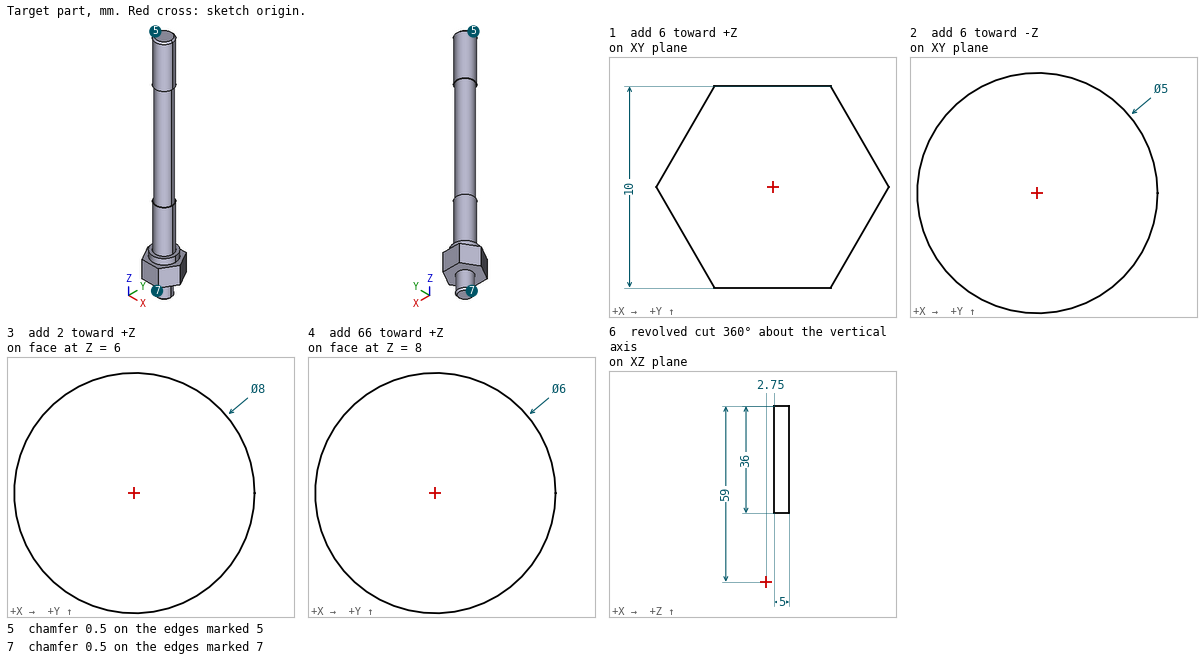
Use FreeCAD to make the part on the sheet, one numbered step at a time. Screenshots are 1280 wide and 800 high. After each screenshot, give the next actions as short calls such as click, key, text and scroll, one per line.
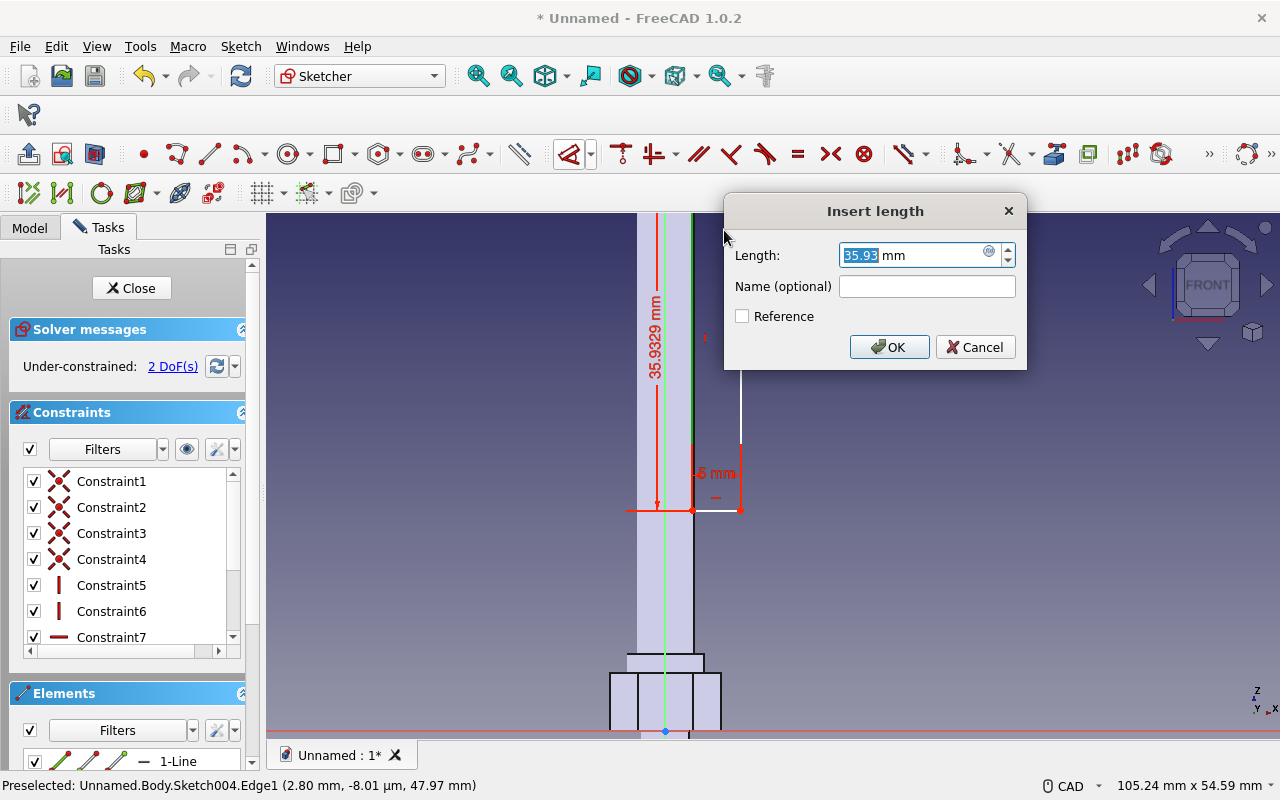
text(36)
key(Return)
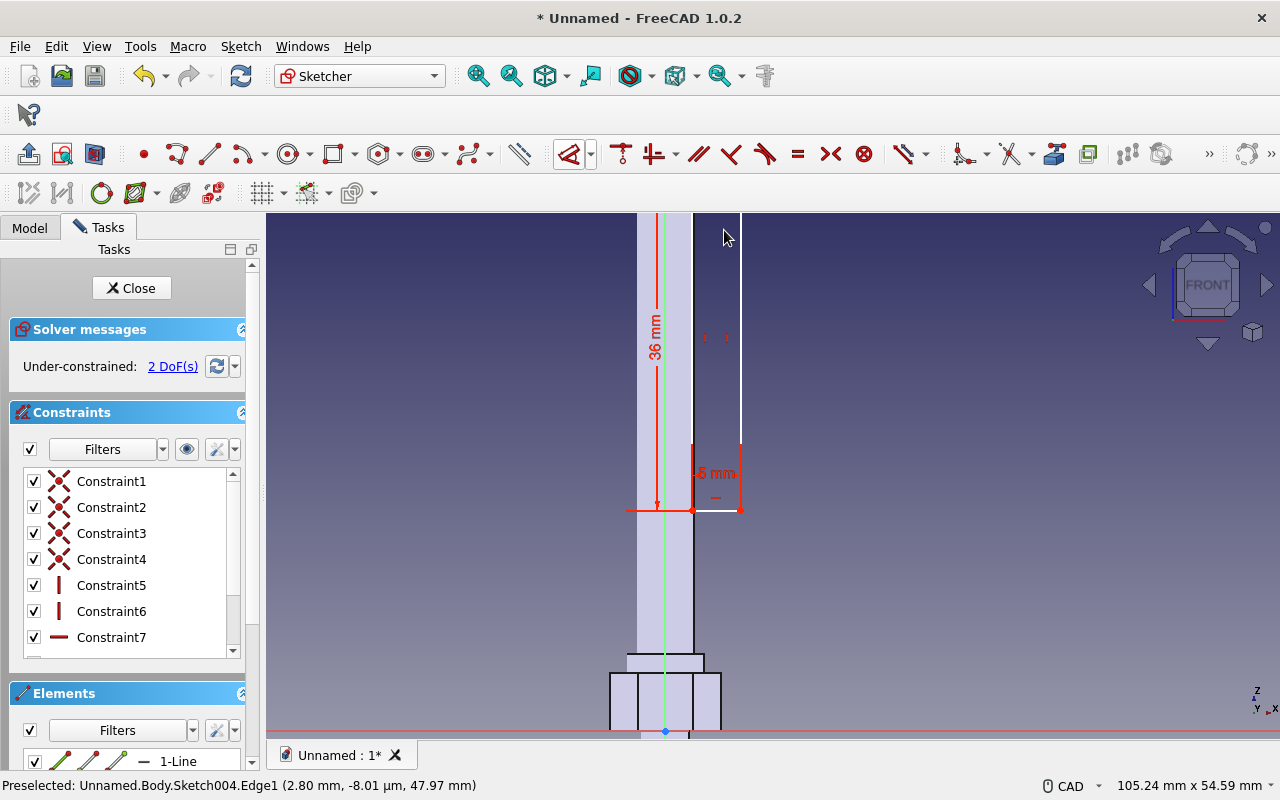
scroll(707, 511, down, 3)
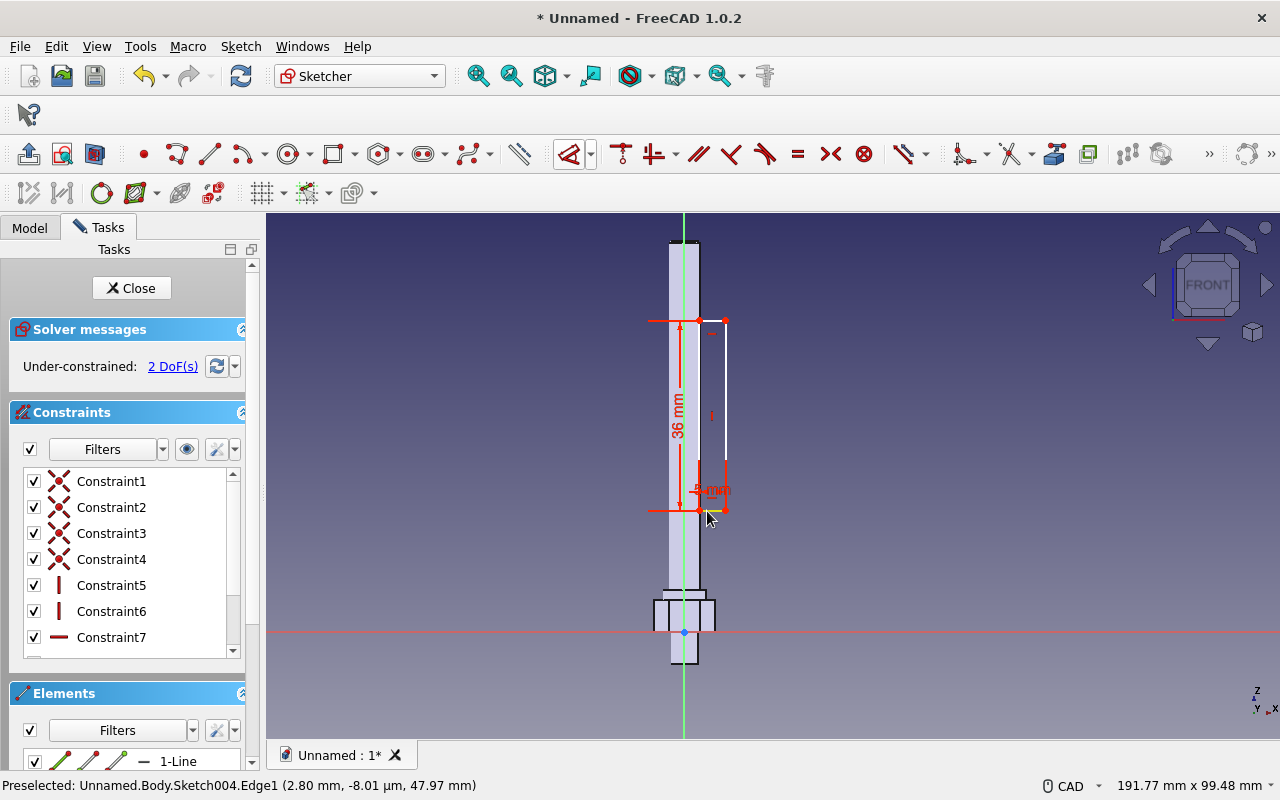
click(699, 321)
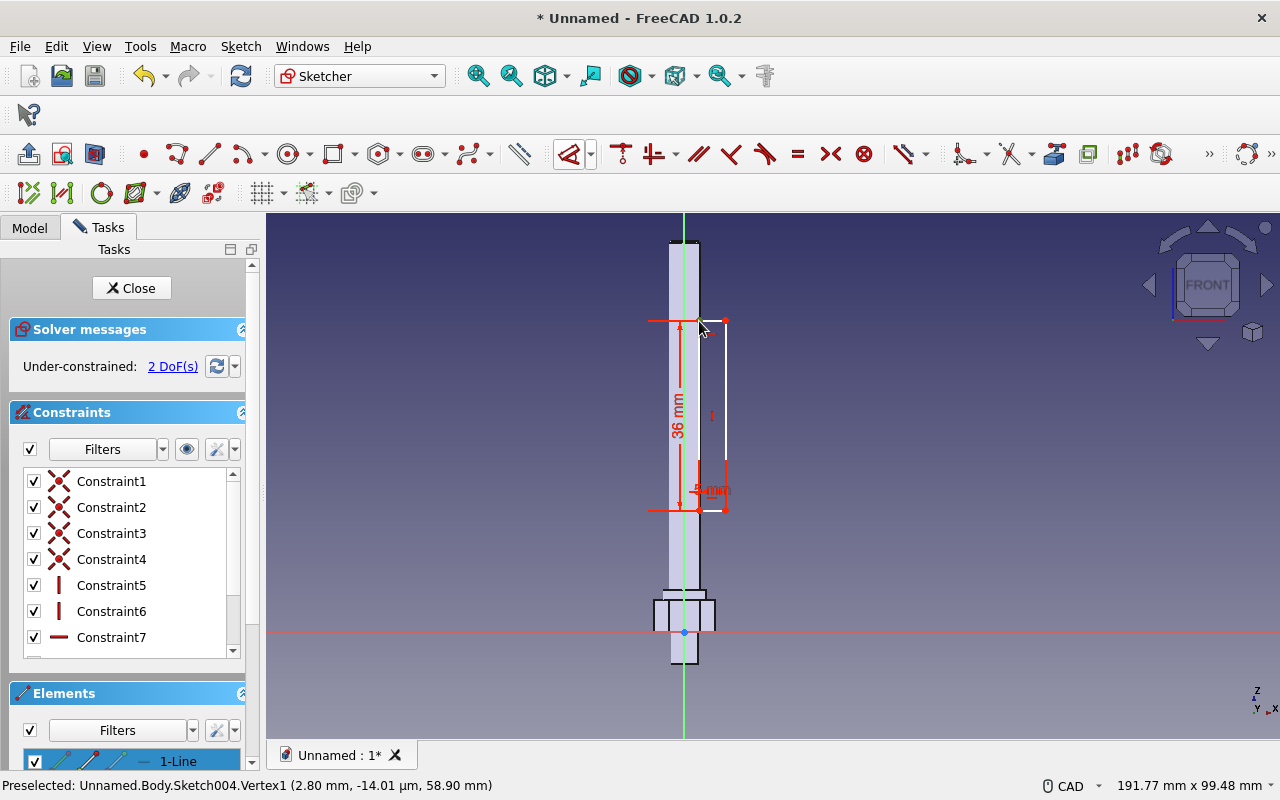
key(i)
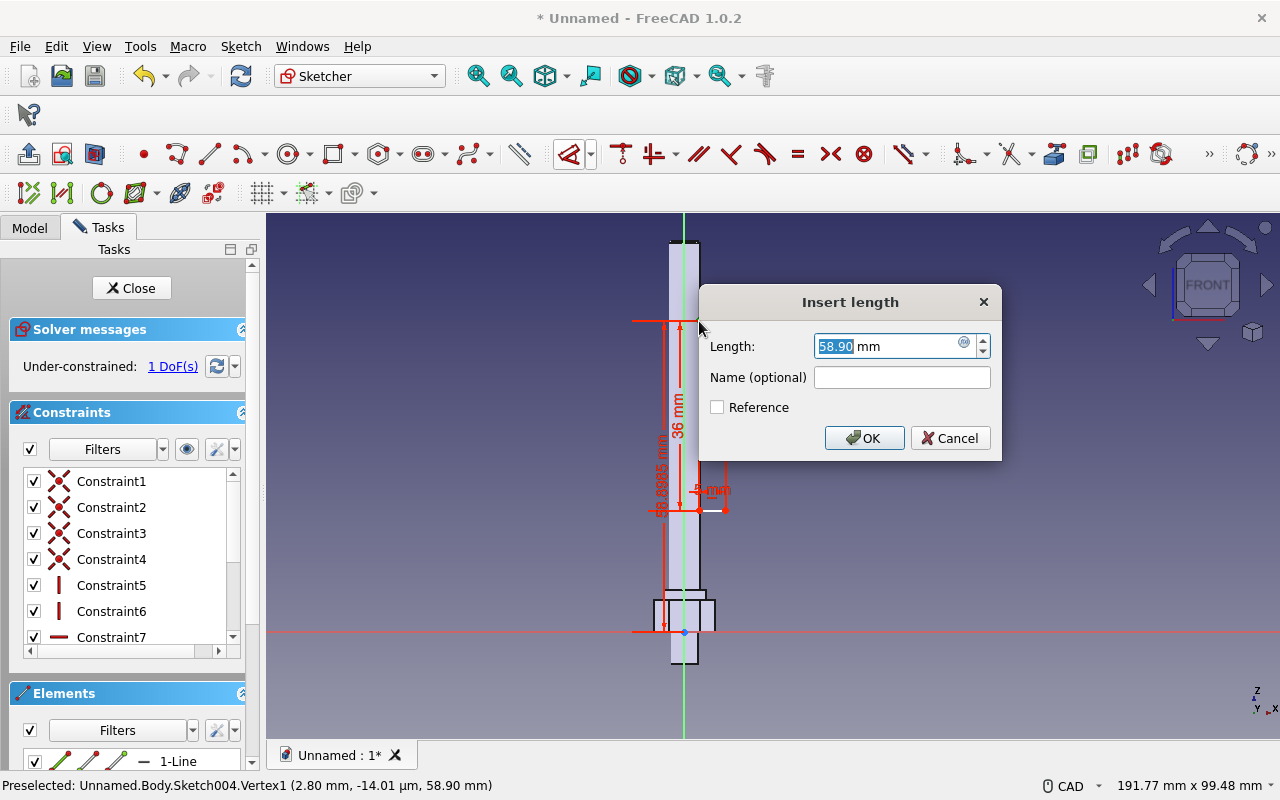
text(59)
key(Return)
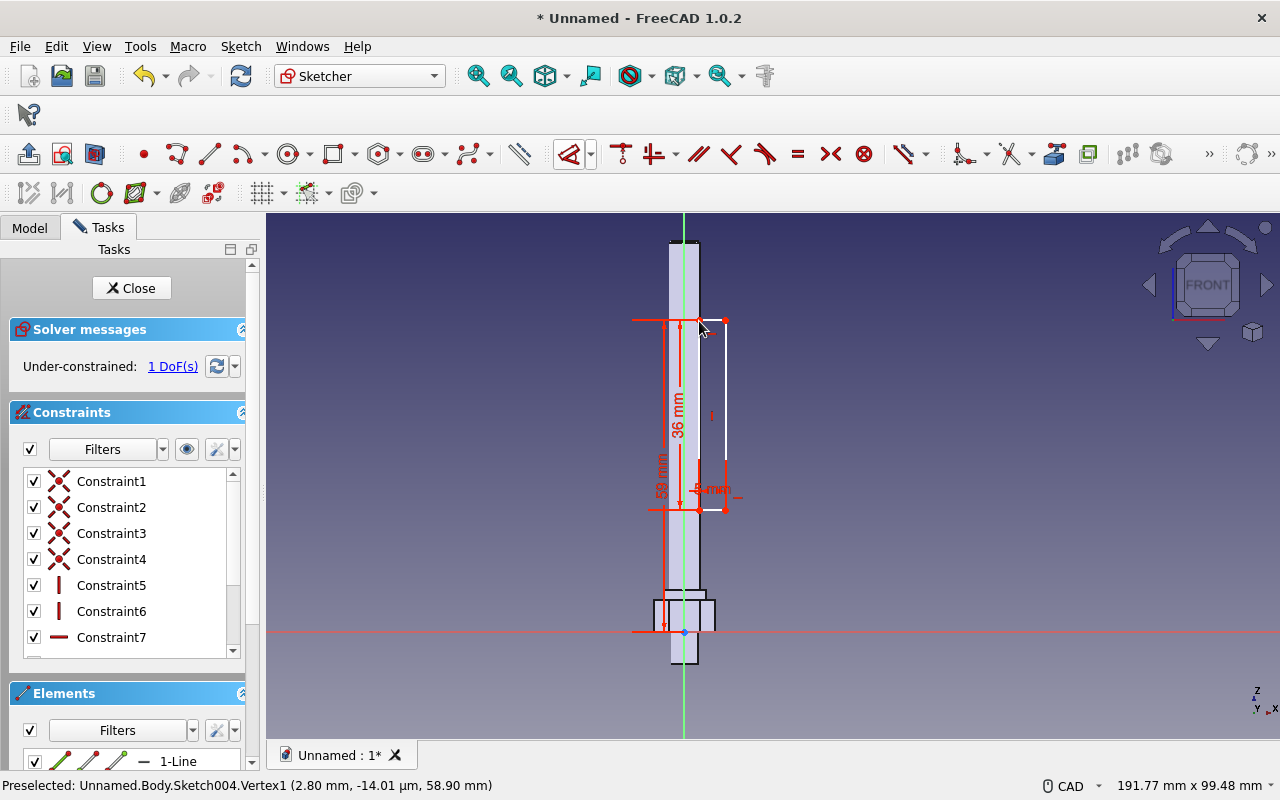
scroll(699, 320, up, 6)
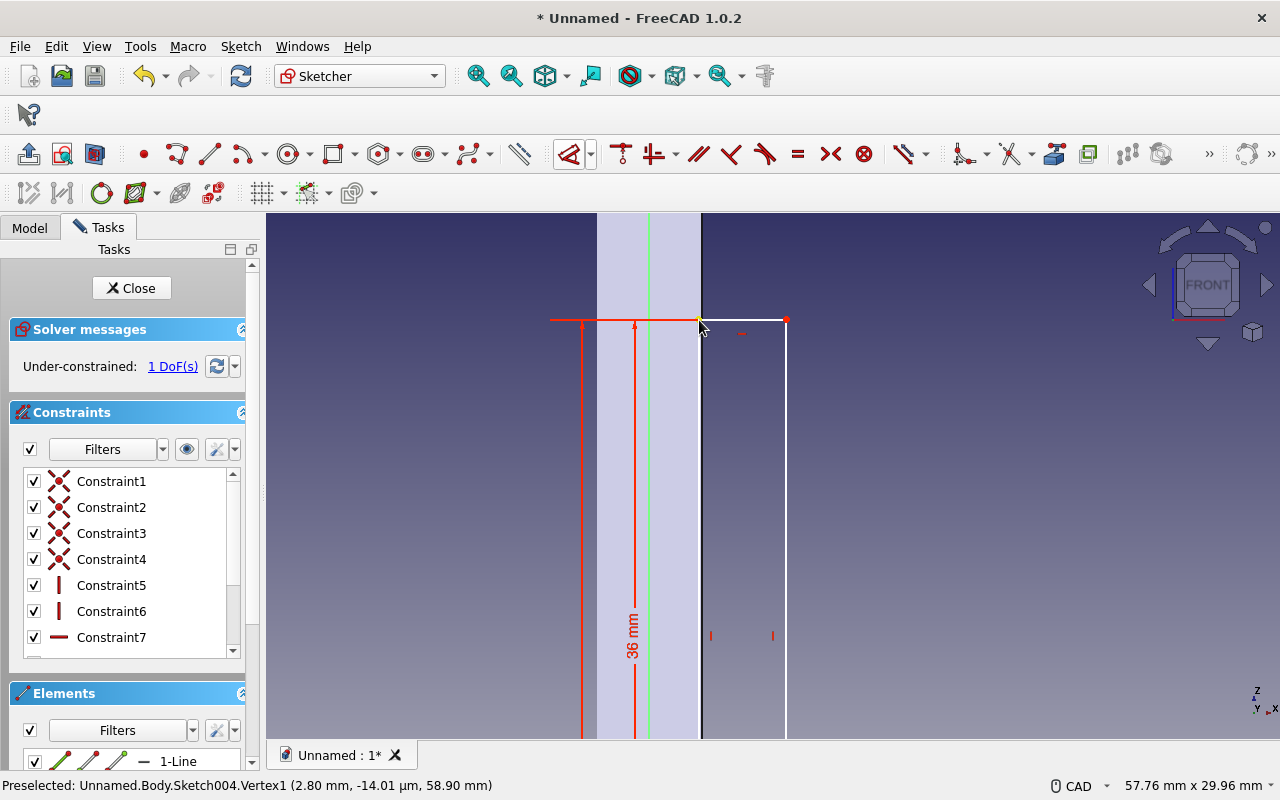
click(699, 320)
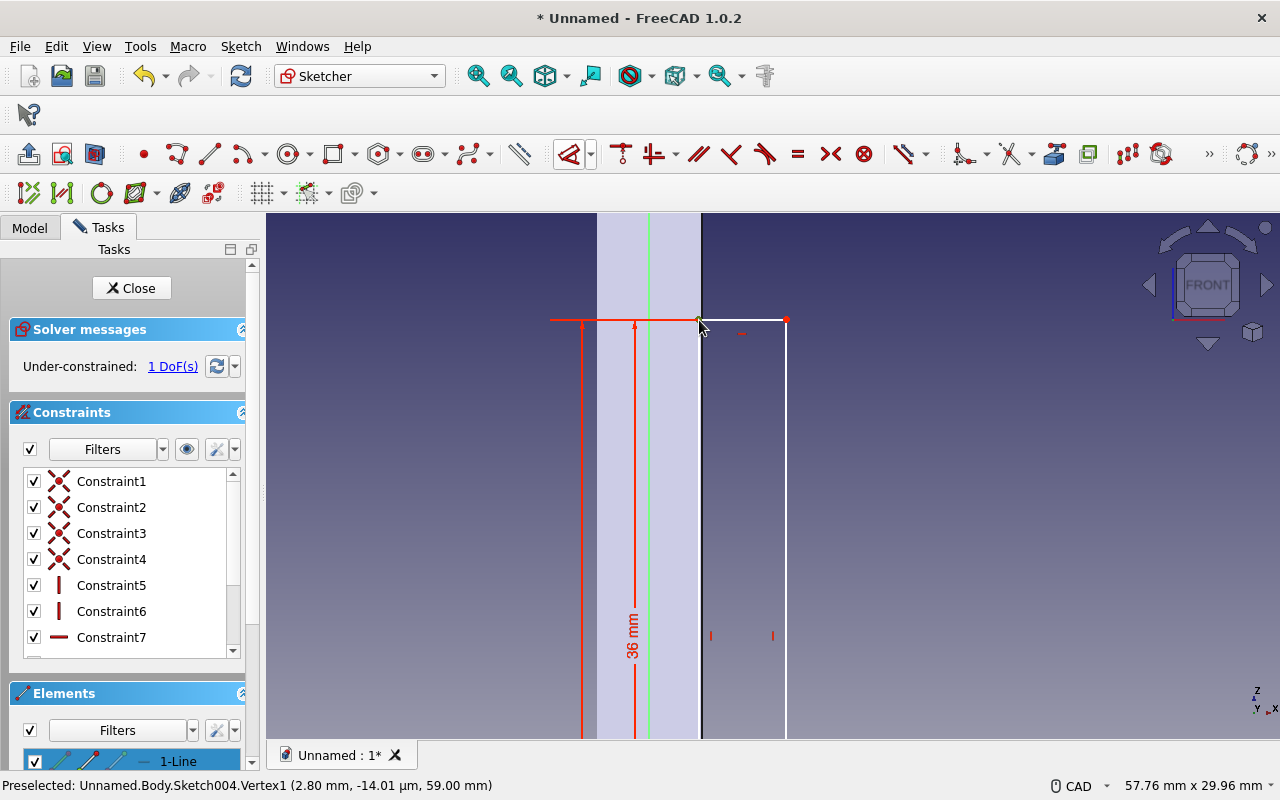
key(l)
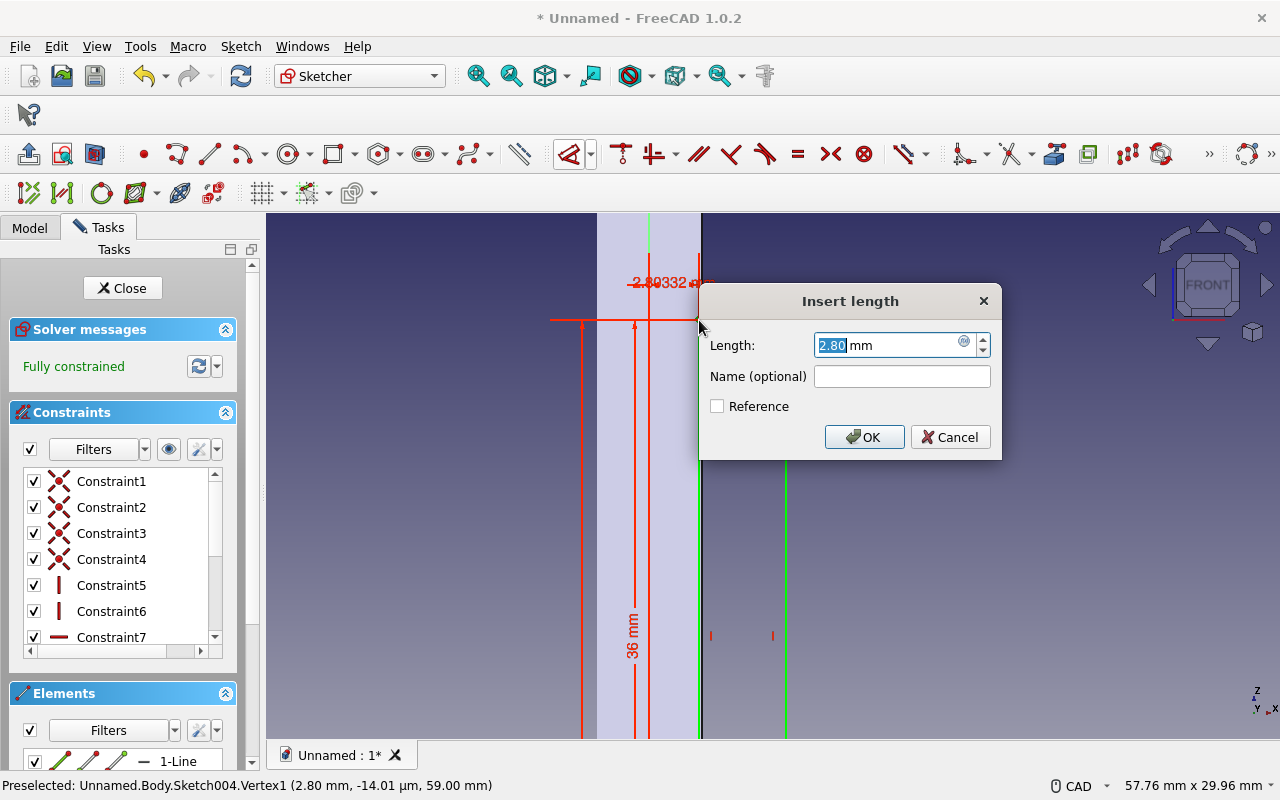
text(2.75)
key(Return)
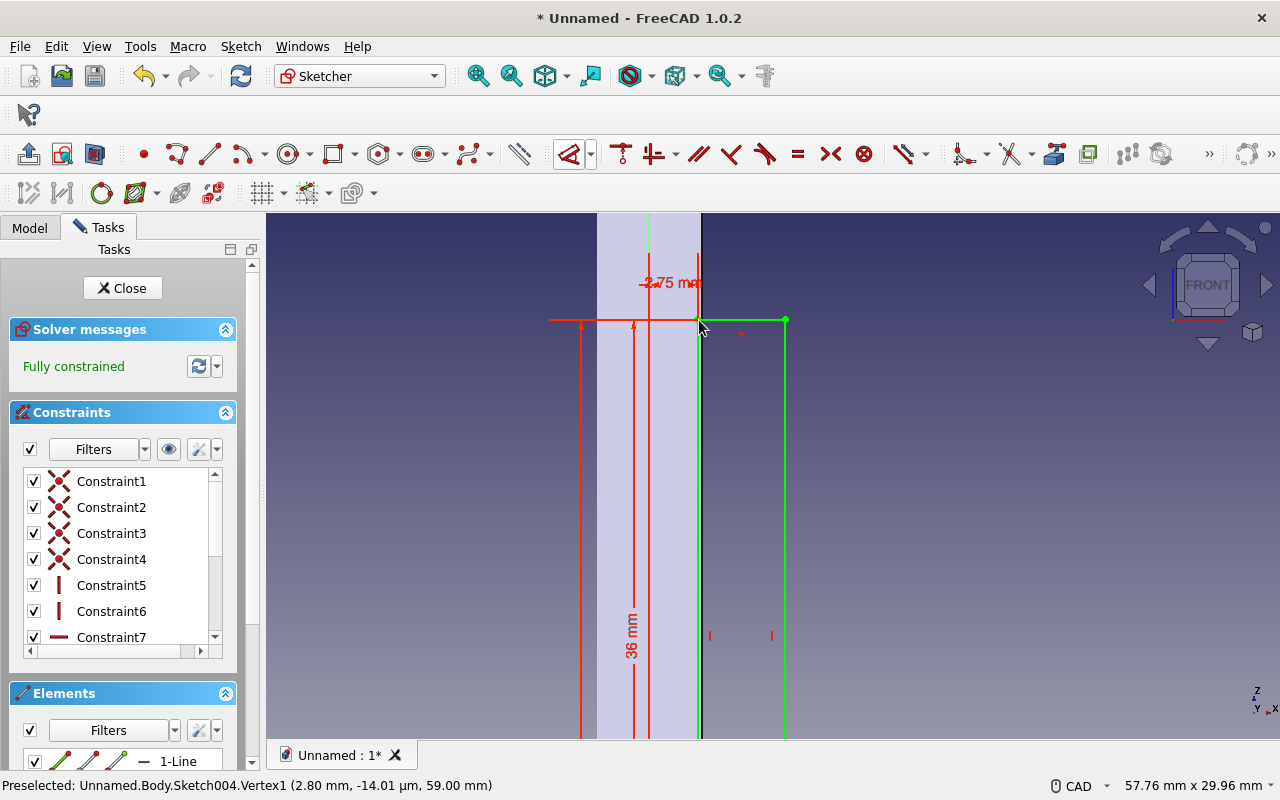
click(123, 288)